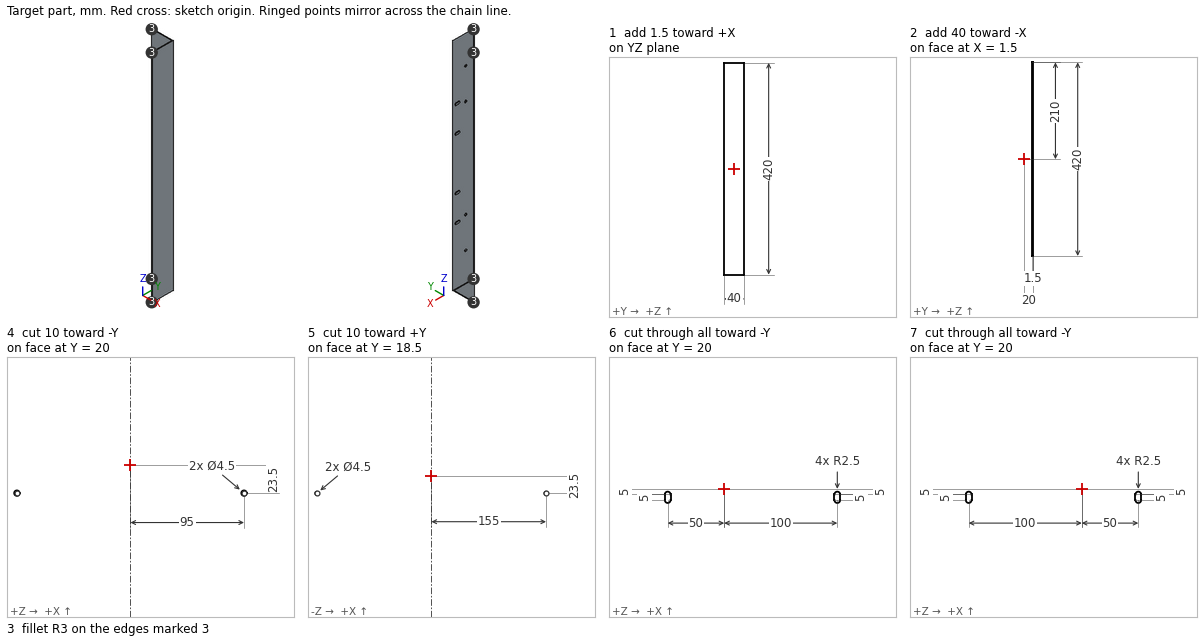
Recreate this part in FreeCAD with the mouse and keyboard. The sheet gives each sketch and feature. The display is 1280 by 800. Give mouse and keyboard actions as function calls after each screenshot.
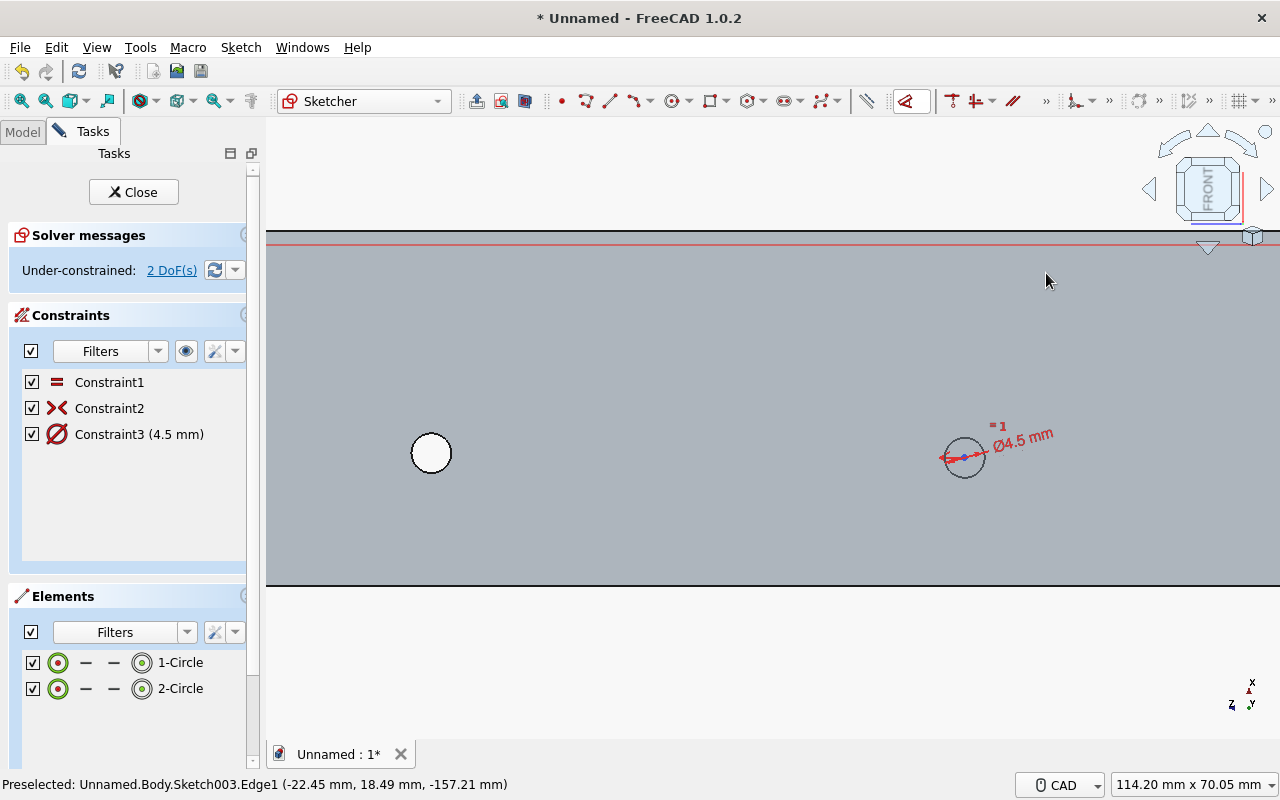
scroll(987, 445, down, 8)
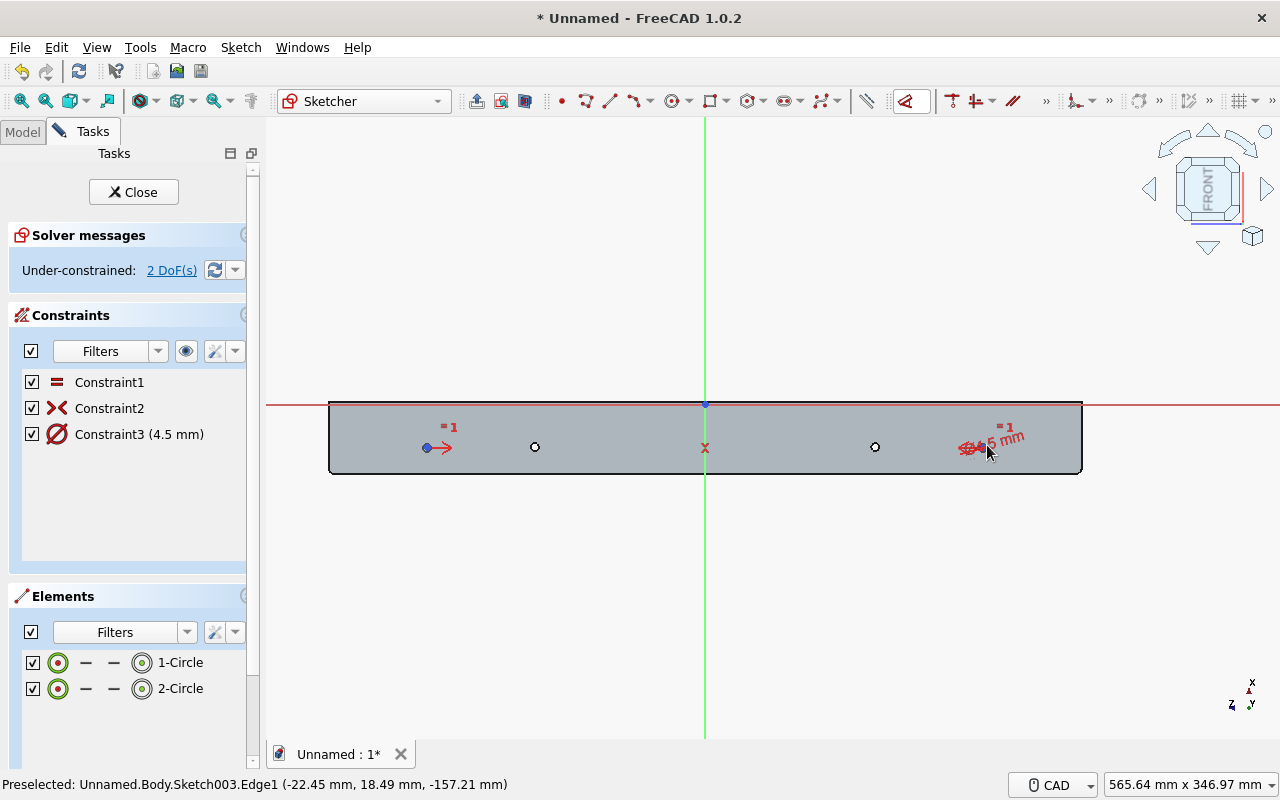
click(983, 448)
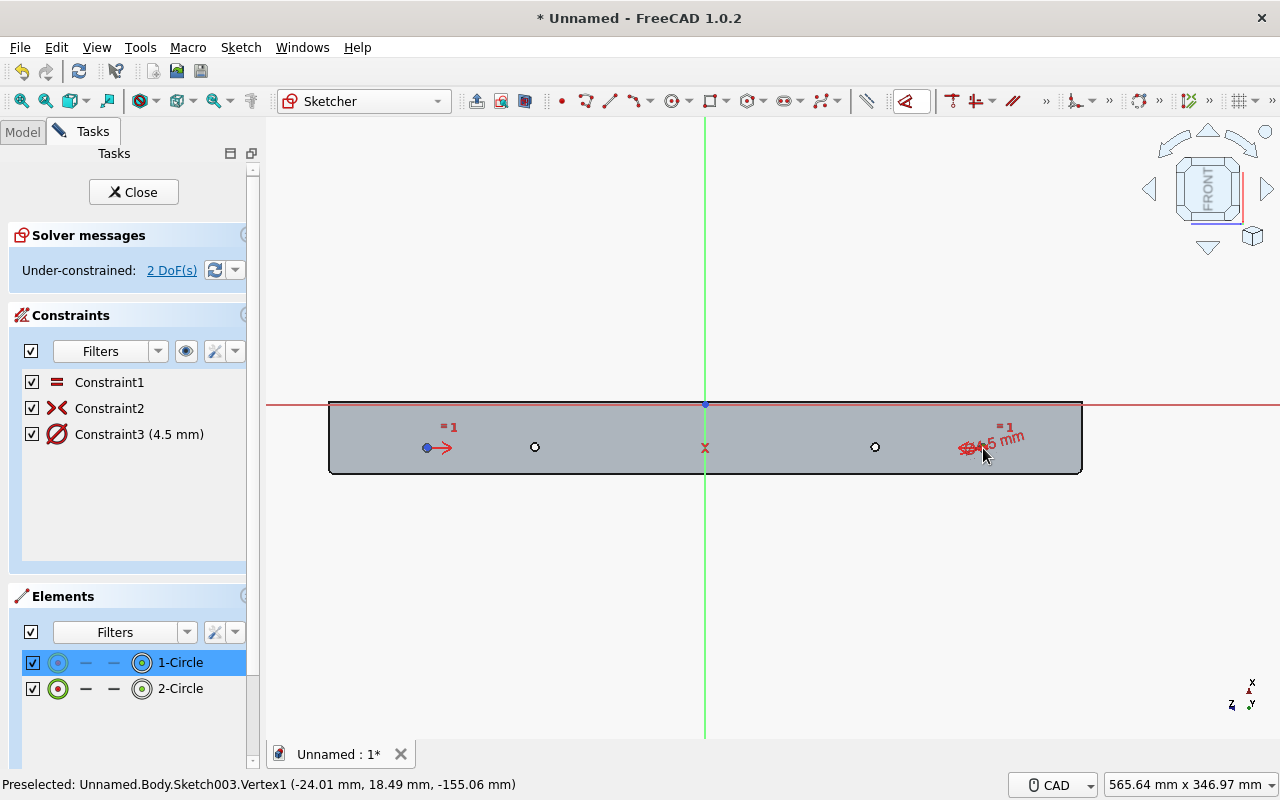
key(l)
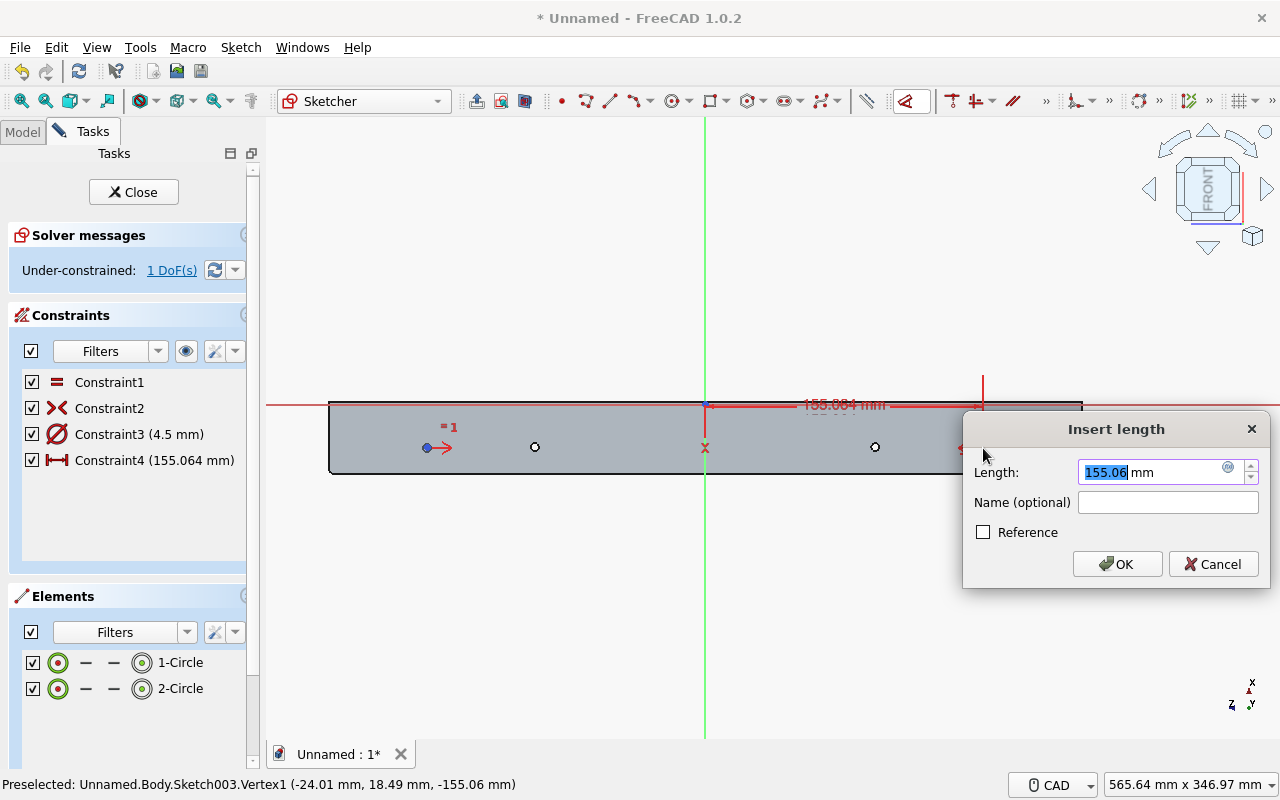
text(155)
key(Return)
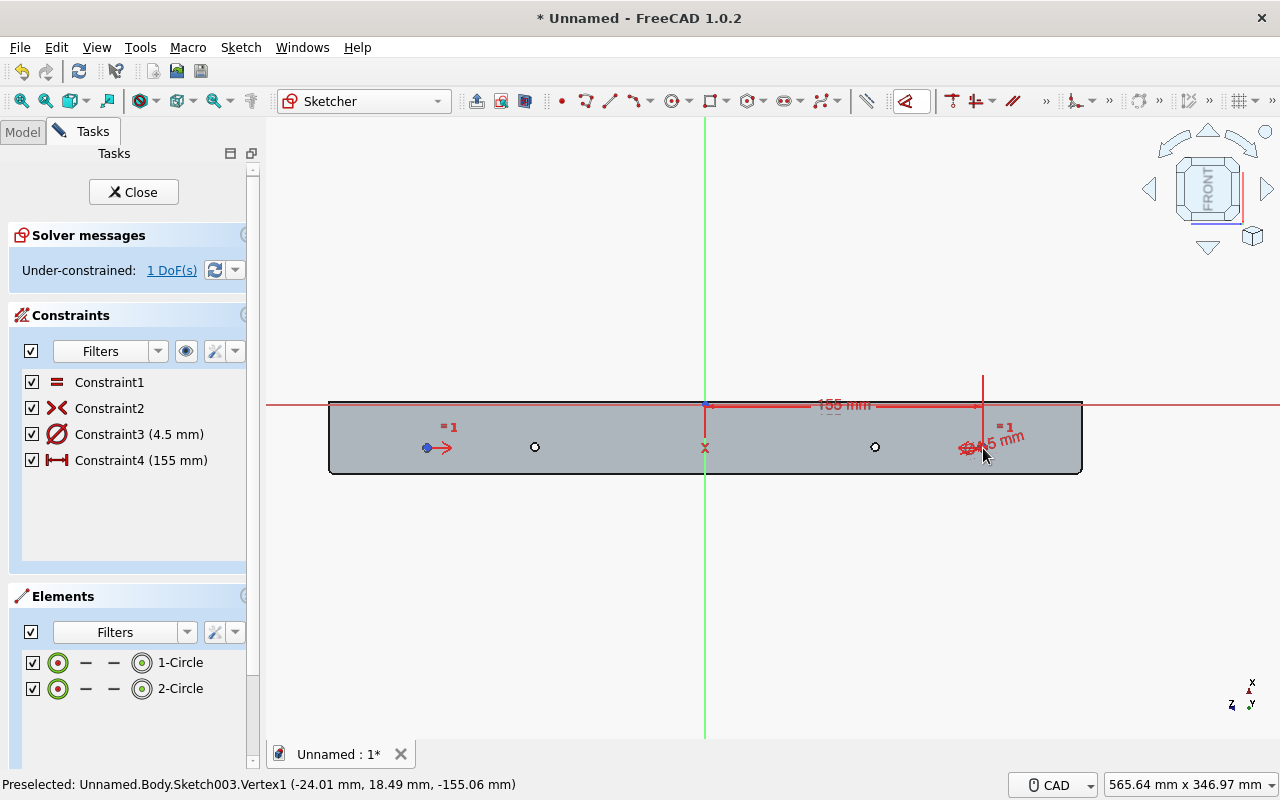
click(983, 448)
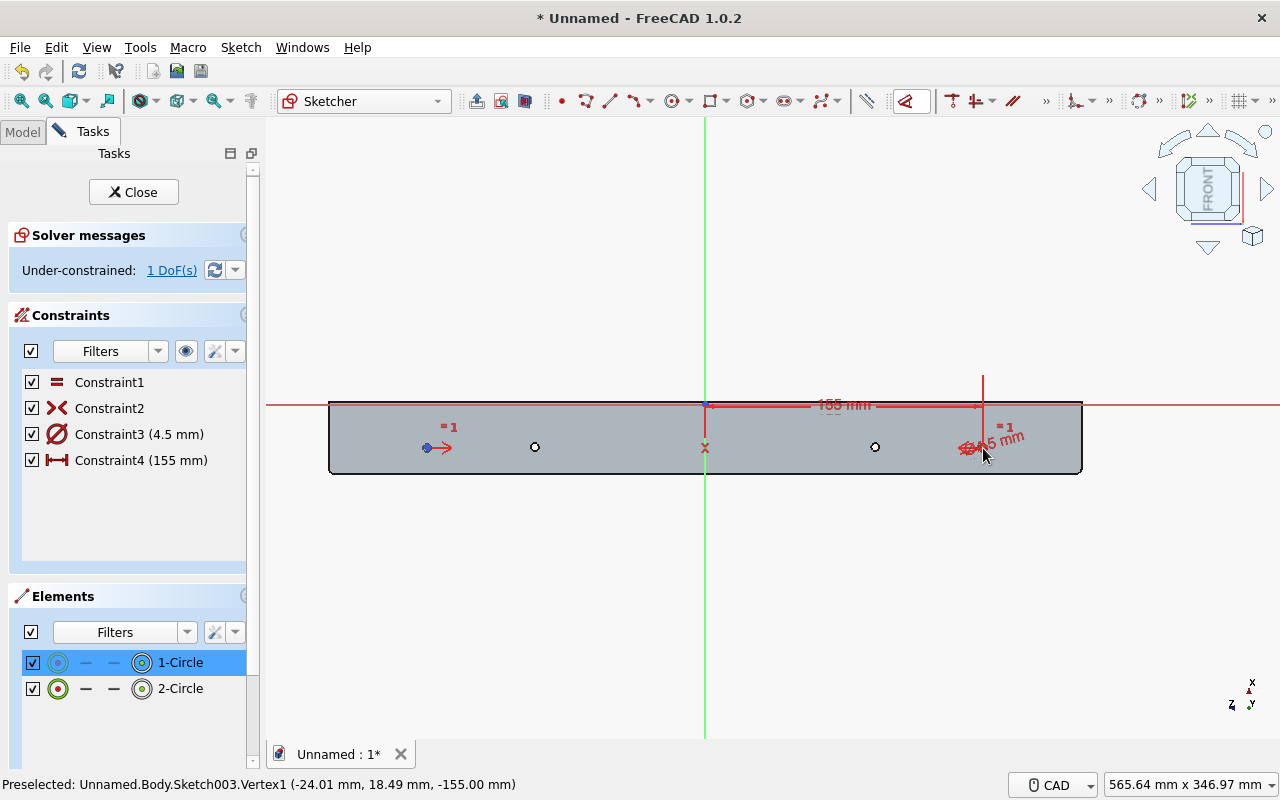
key(i)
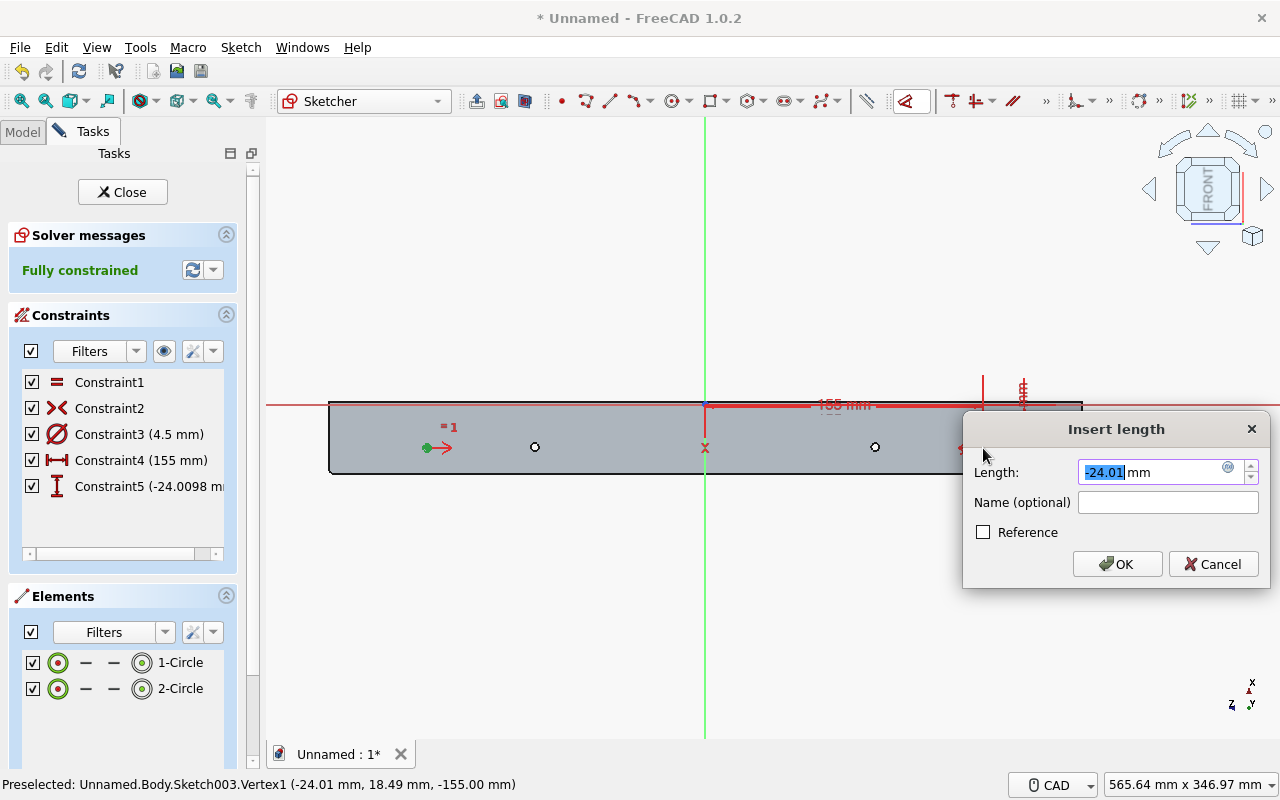
text(-23.5)
key(Return)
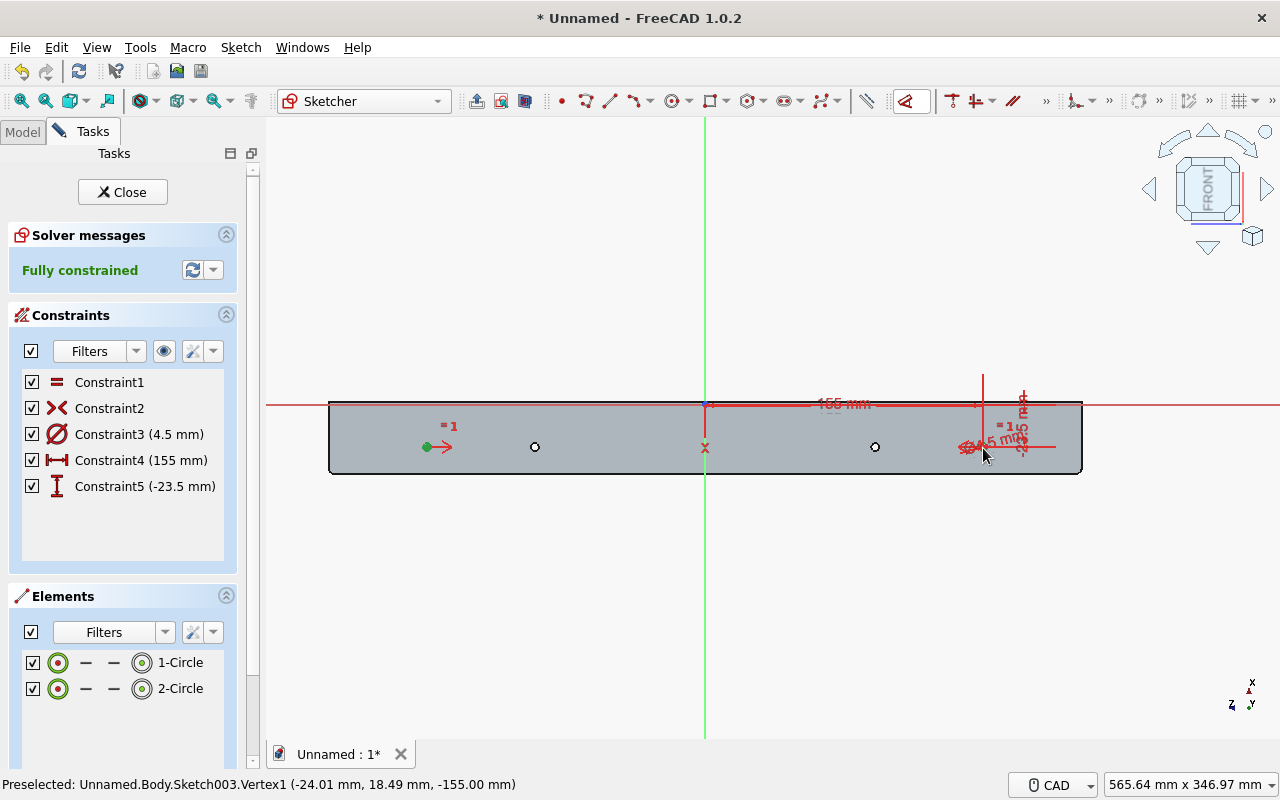
click(123, 192)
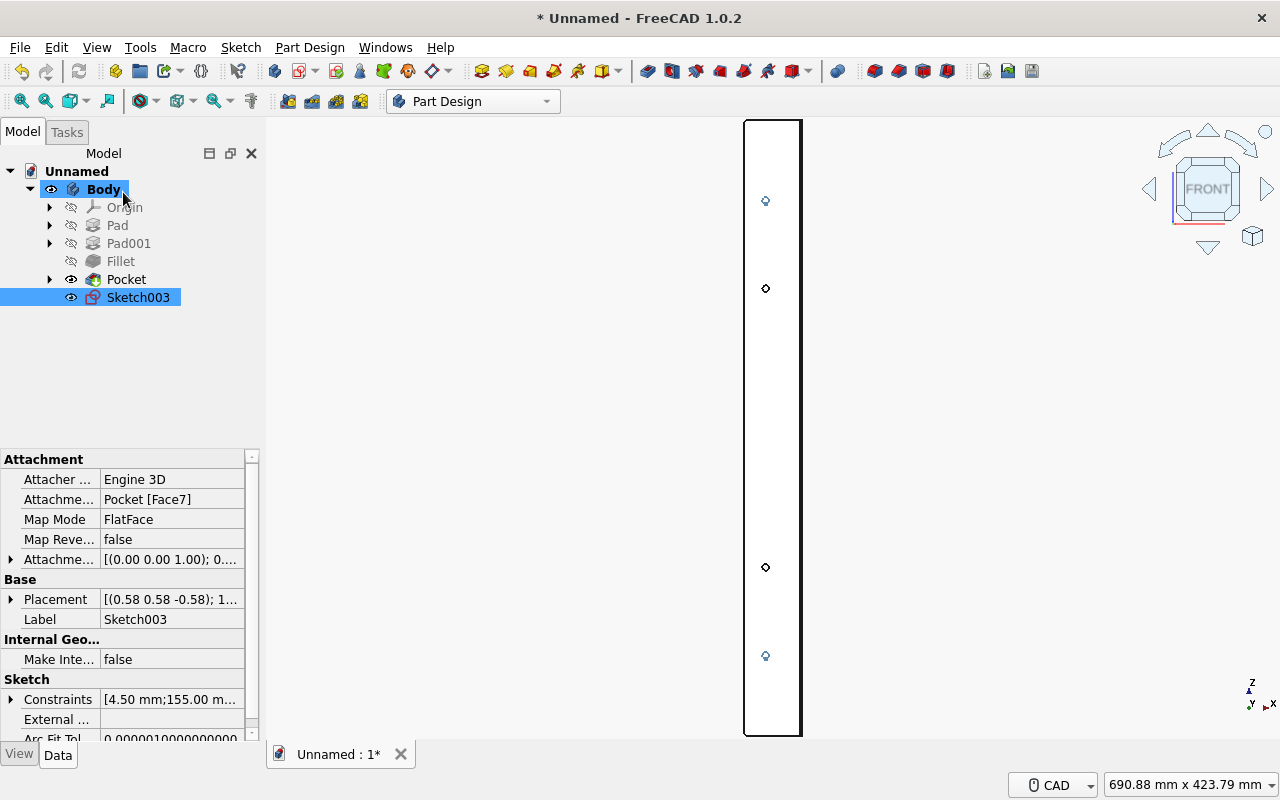
click(648, 72)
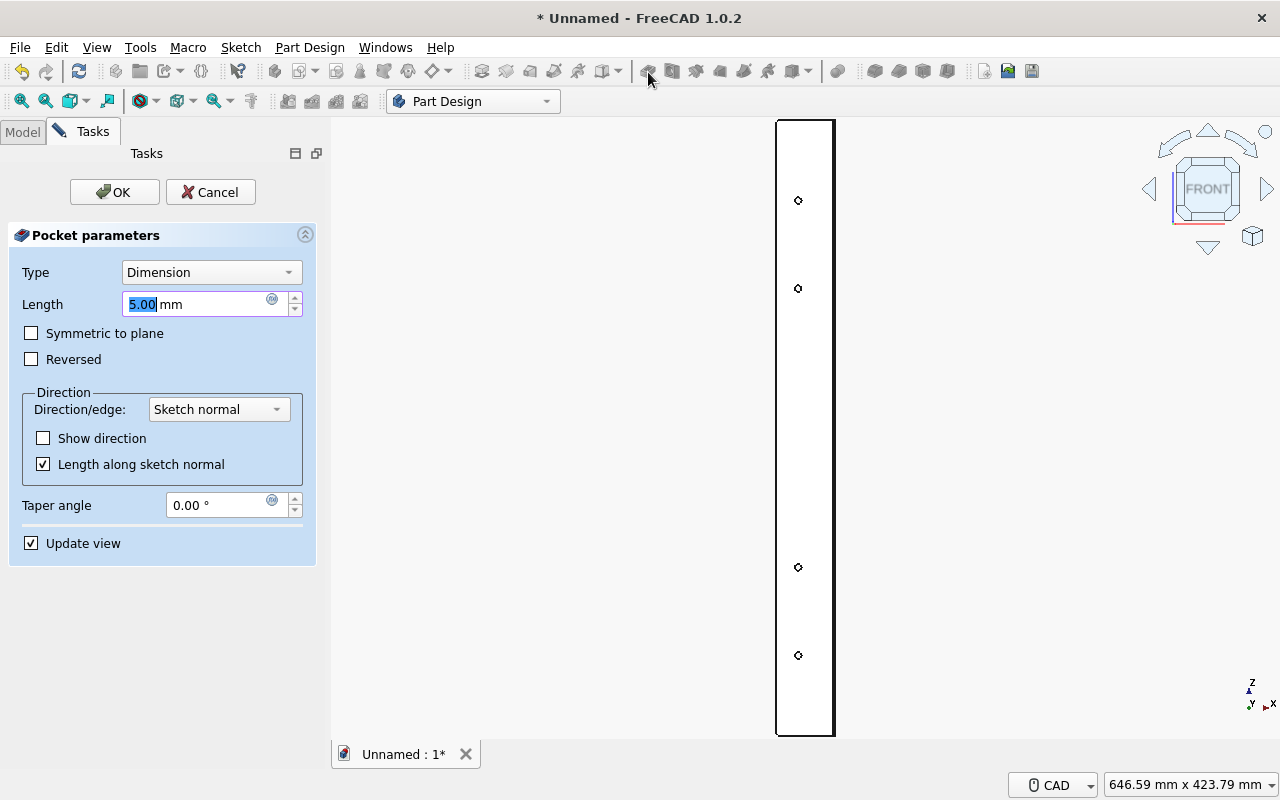
text(10)
key(Tab)